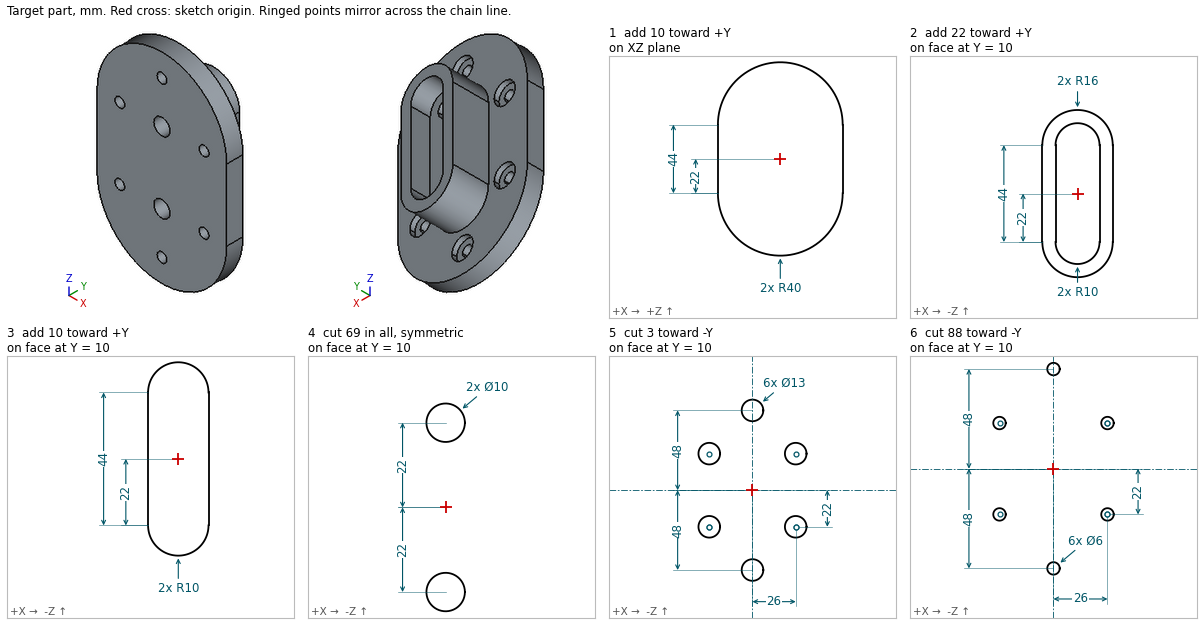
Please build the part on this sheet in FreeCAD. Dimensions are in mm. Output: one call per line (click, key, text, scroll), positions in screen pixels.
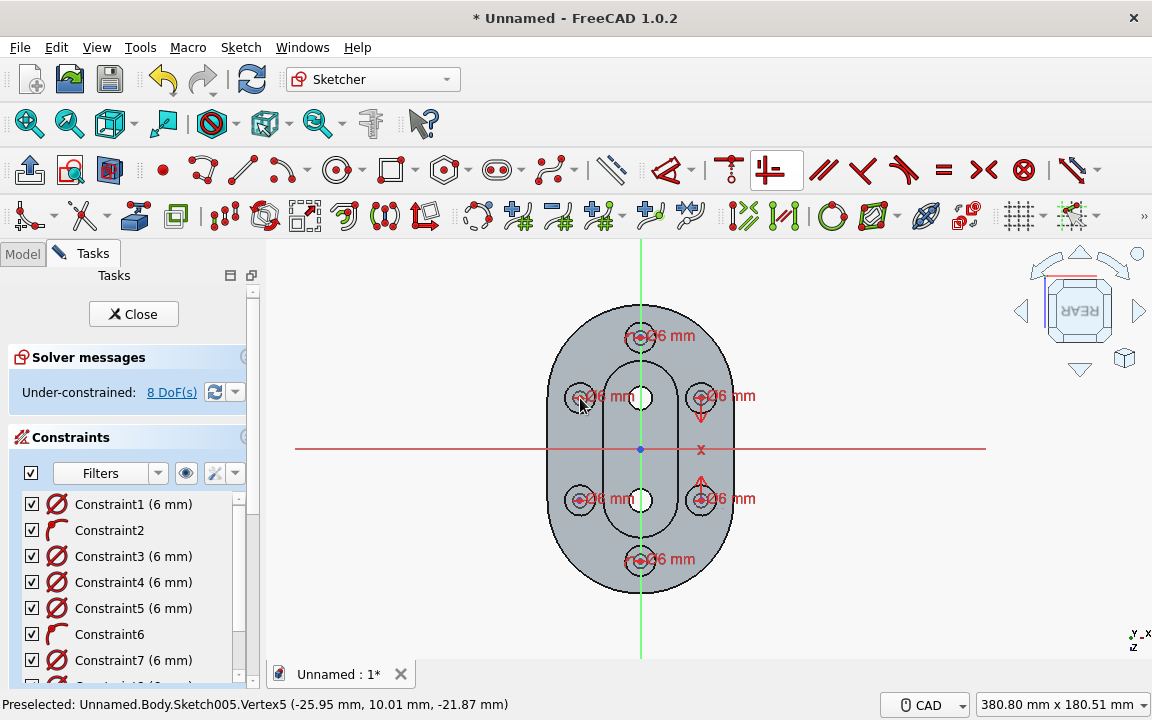
click(641, 605)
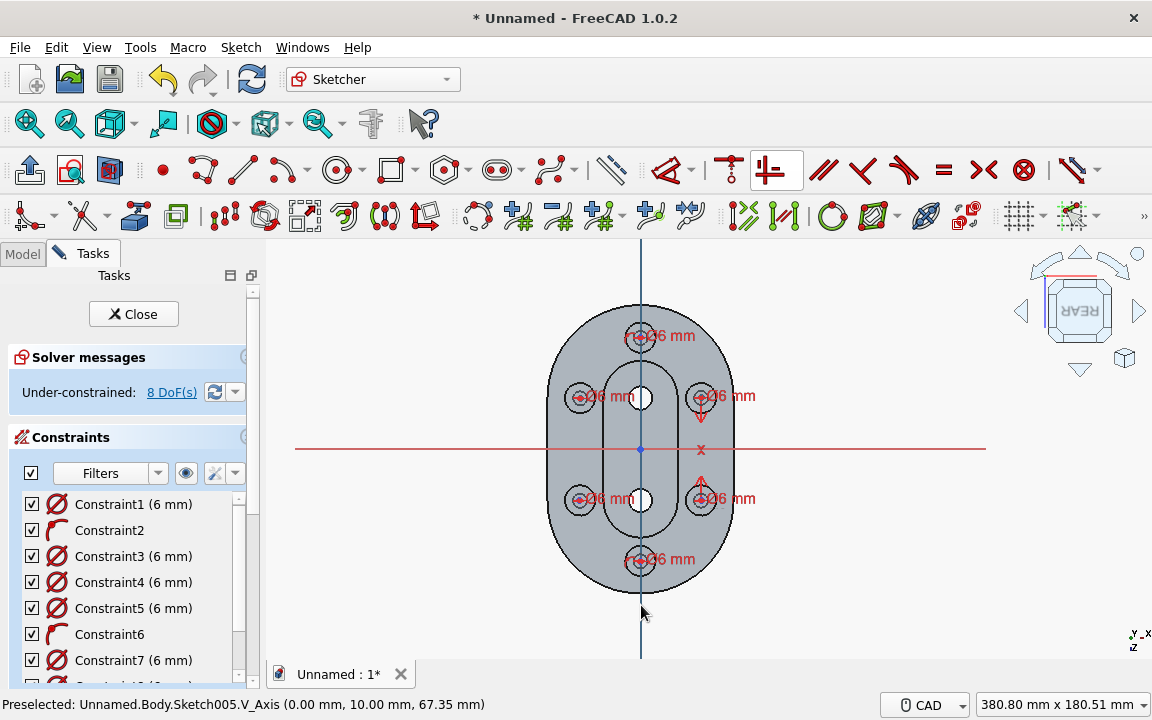
click(984, 170)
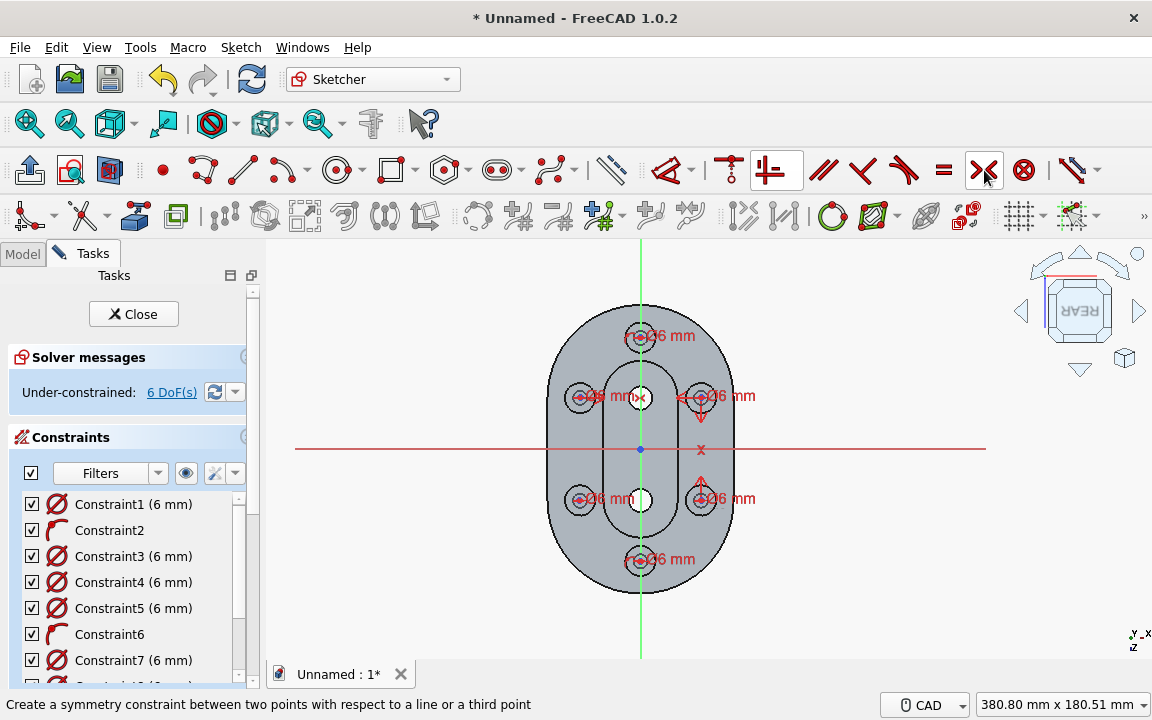
click(701, 501)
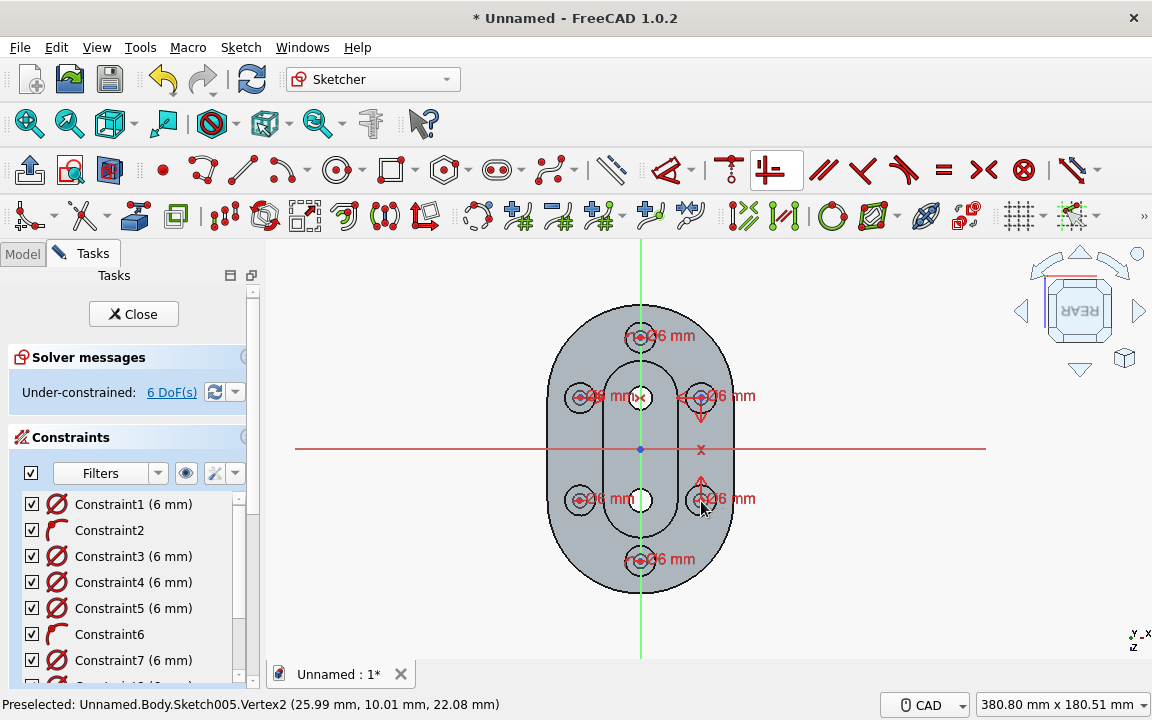
click(580, 501)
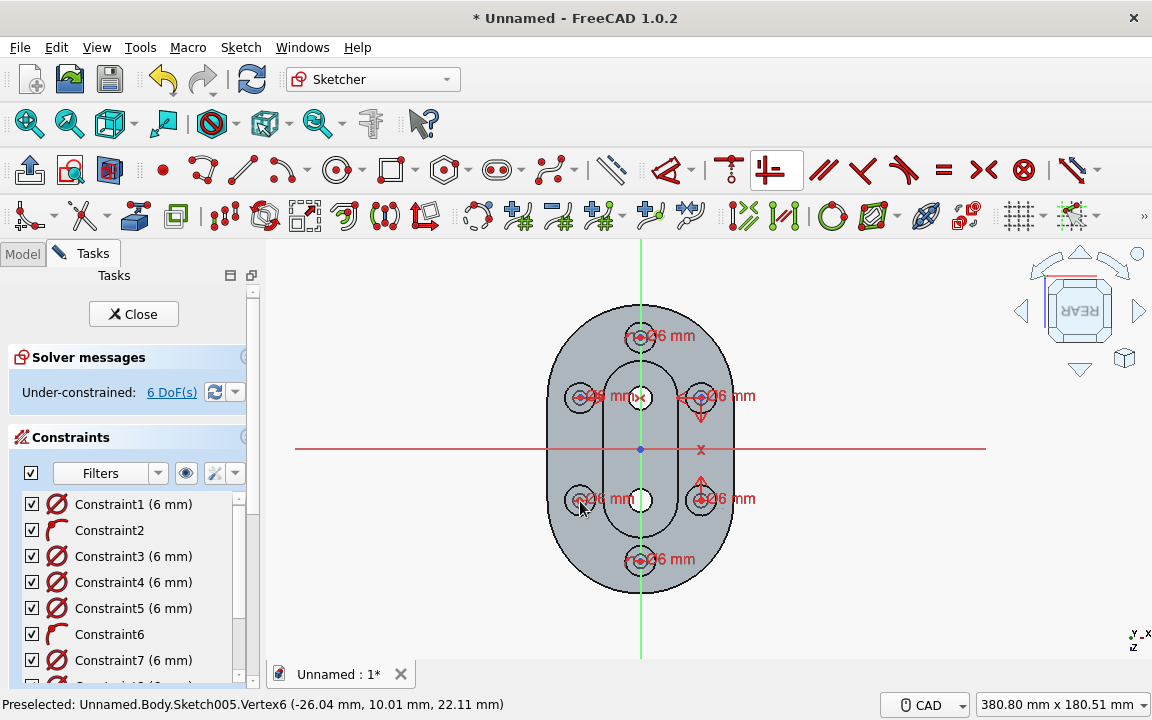
click(641, 605)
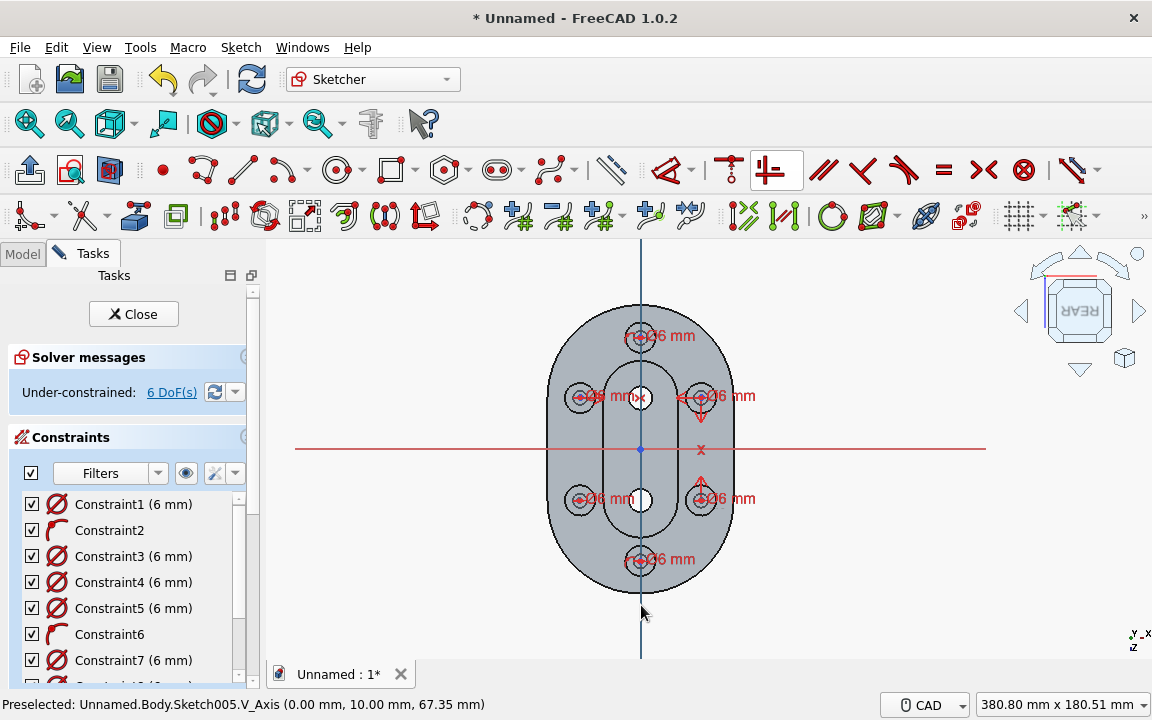
click(984, 170)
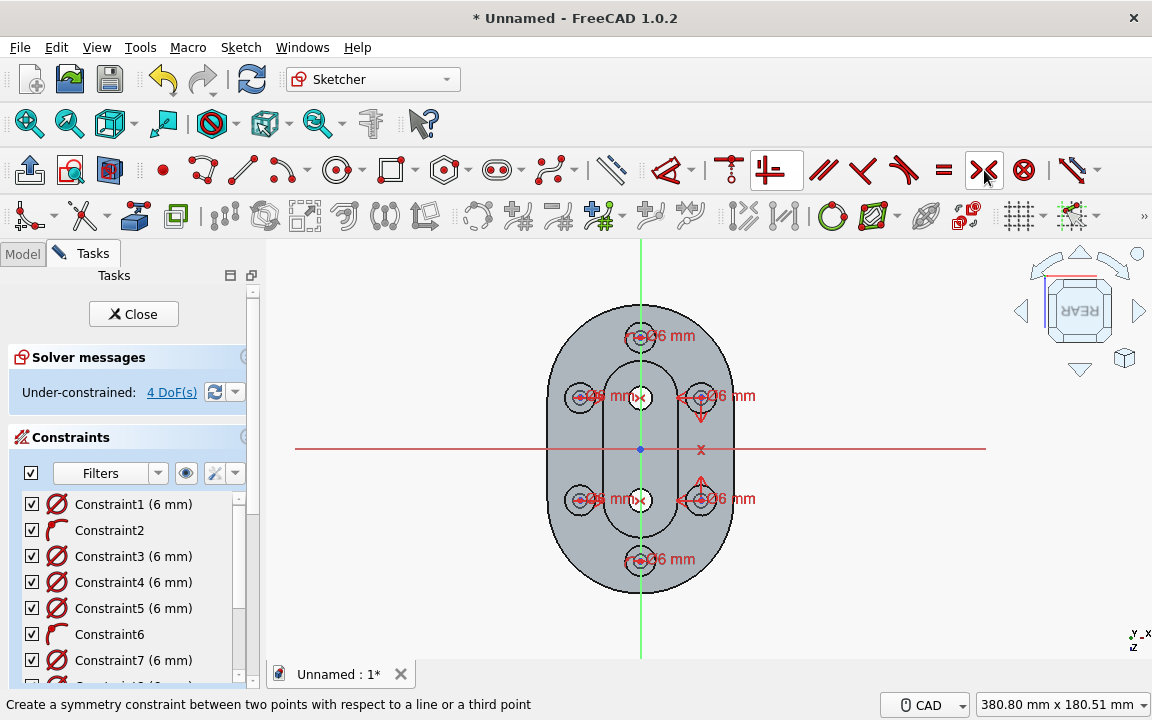
click(666, 170)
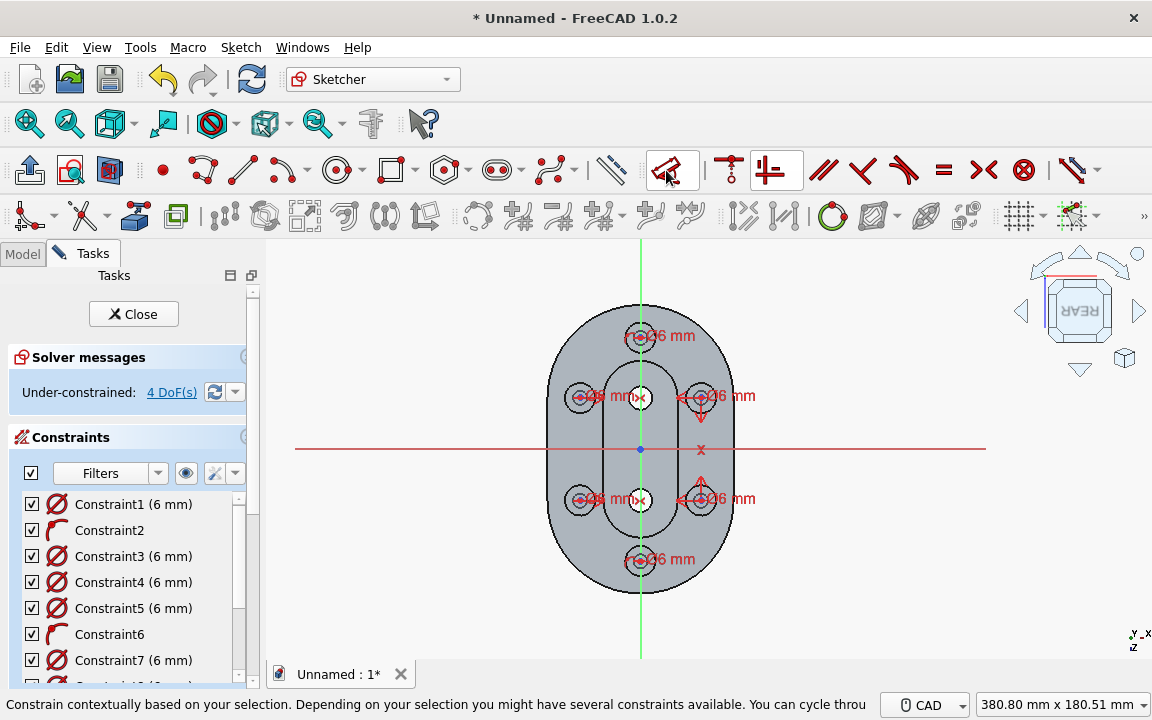
click(641, 561)
click(675, 505)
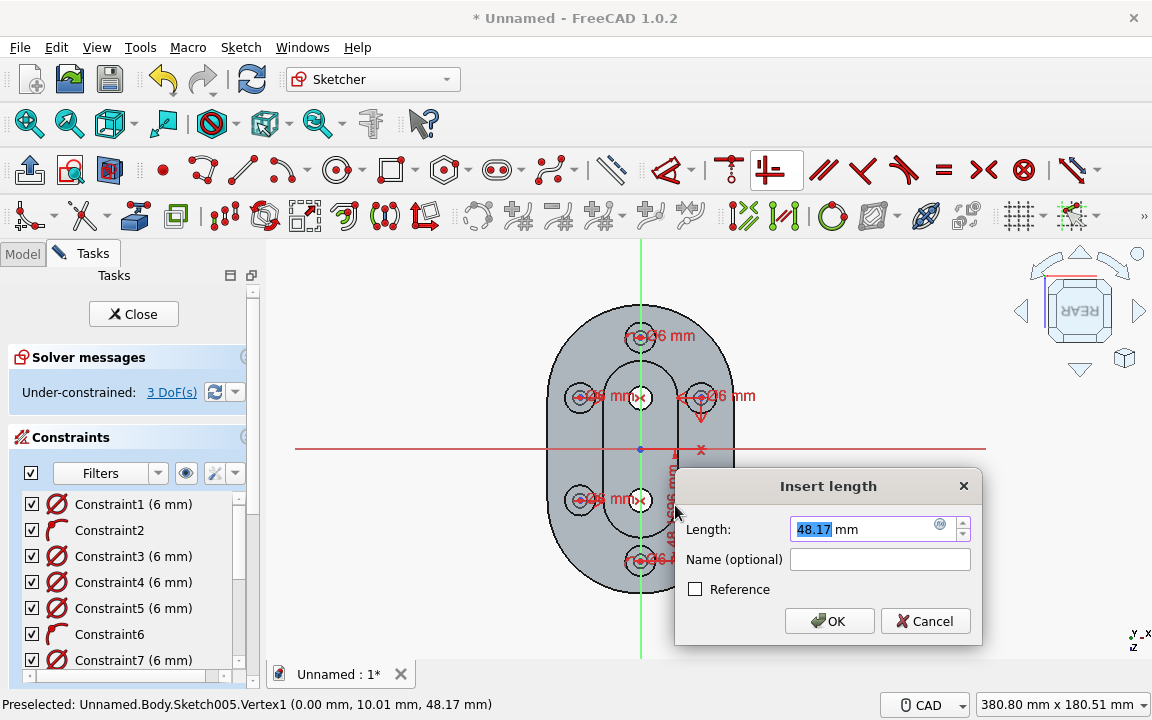
text(48)
key(Return)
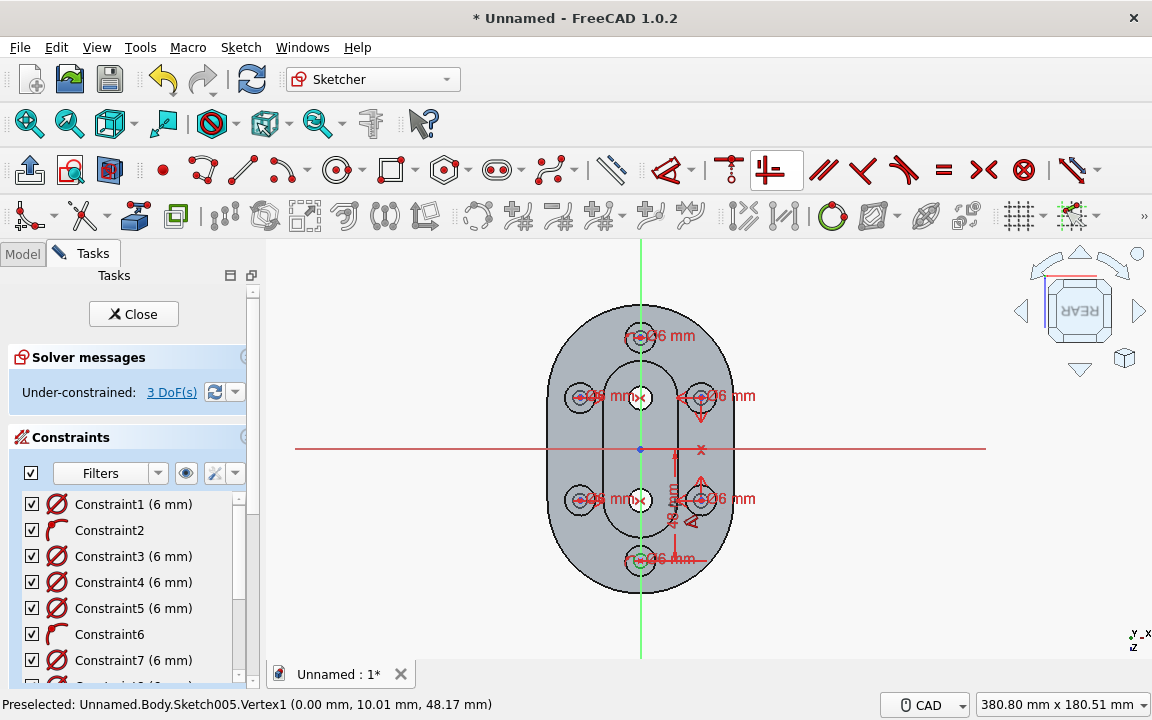
click(701, 501)
click(671, 535)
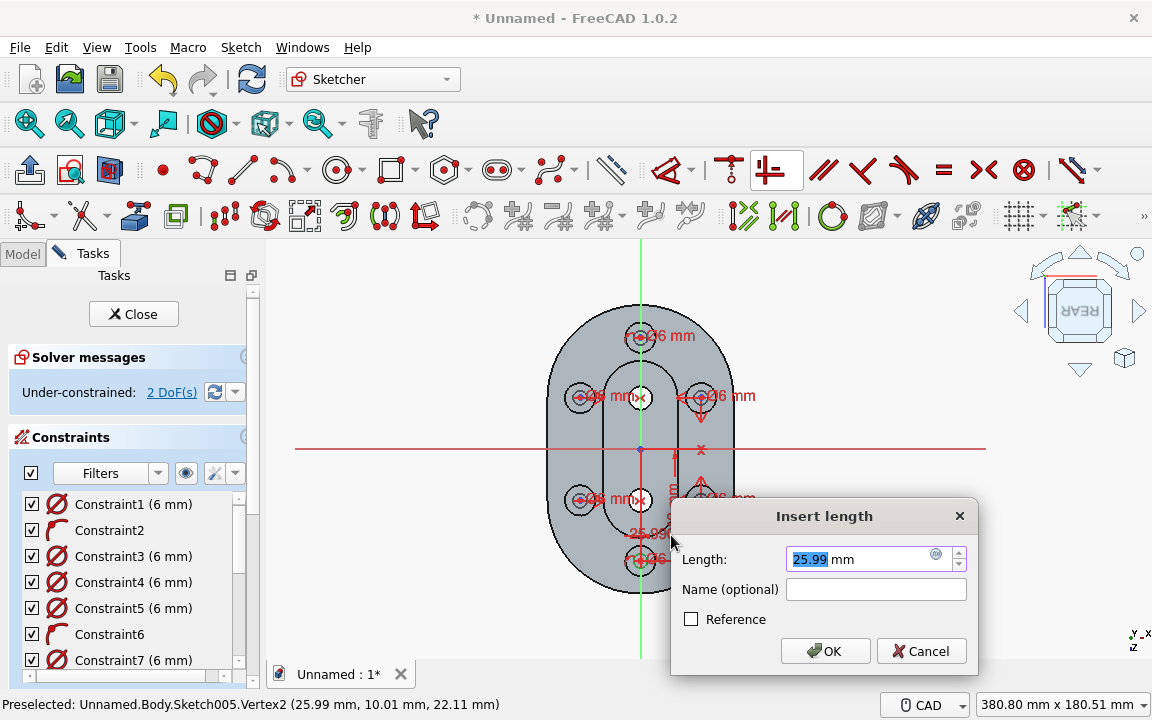
text(26)
key(Return)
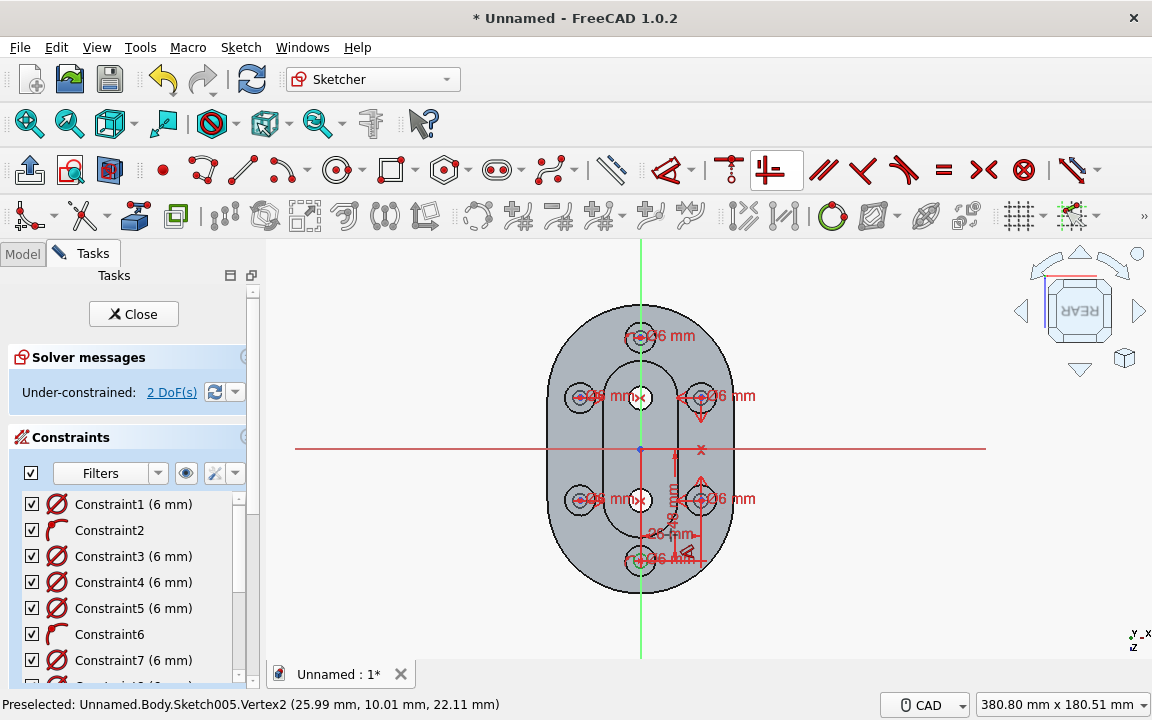
click(701, 501)
click(735, 475)